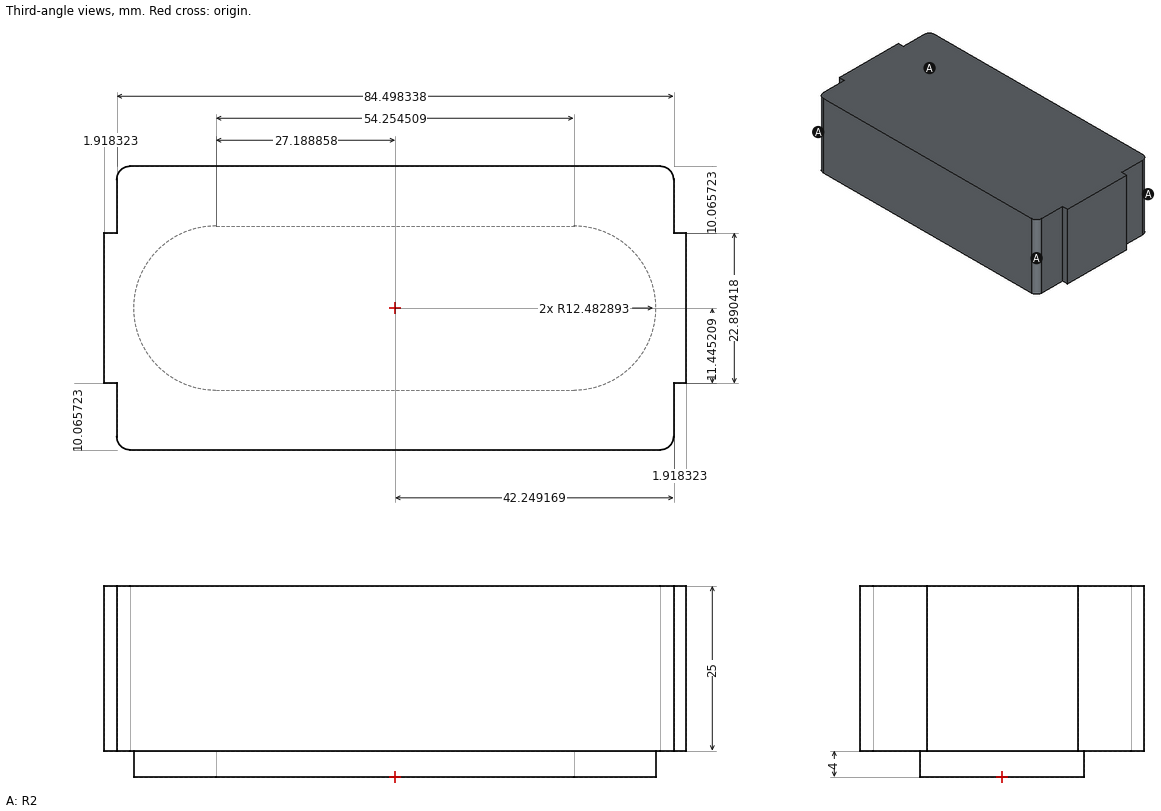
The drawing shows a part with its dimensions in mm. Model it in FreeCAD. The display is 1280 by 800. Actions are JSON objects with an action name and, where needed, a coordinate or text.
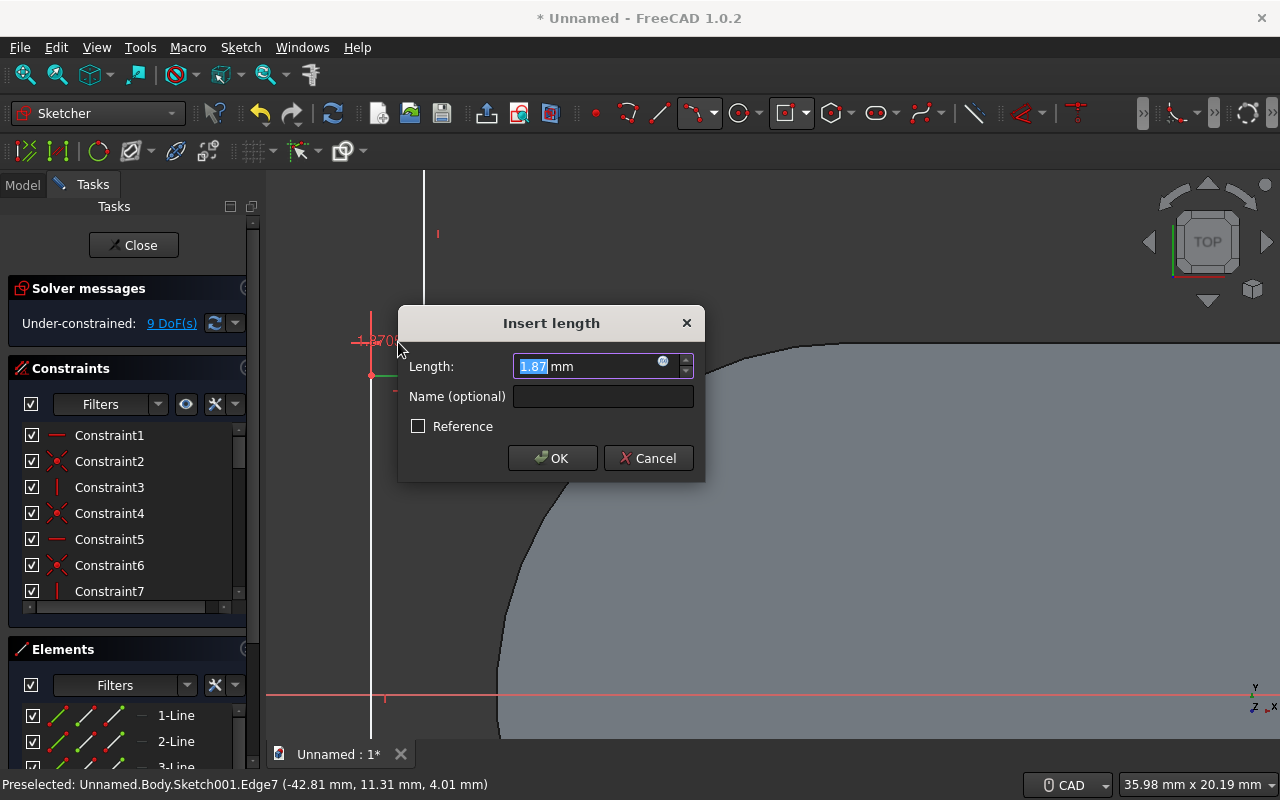
{"action": "type", "text": "1.918323"}
{"action": "key", "text": "Return"}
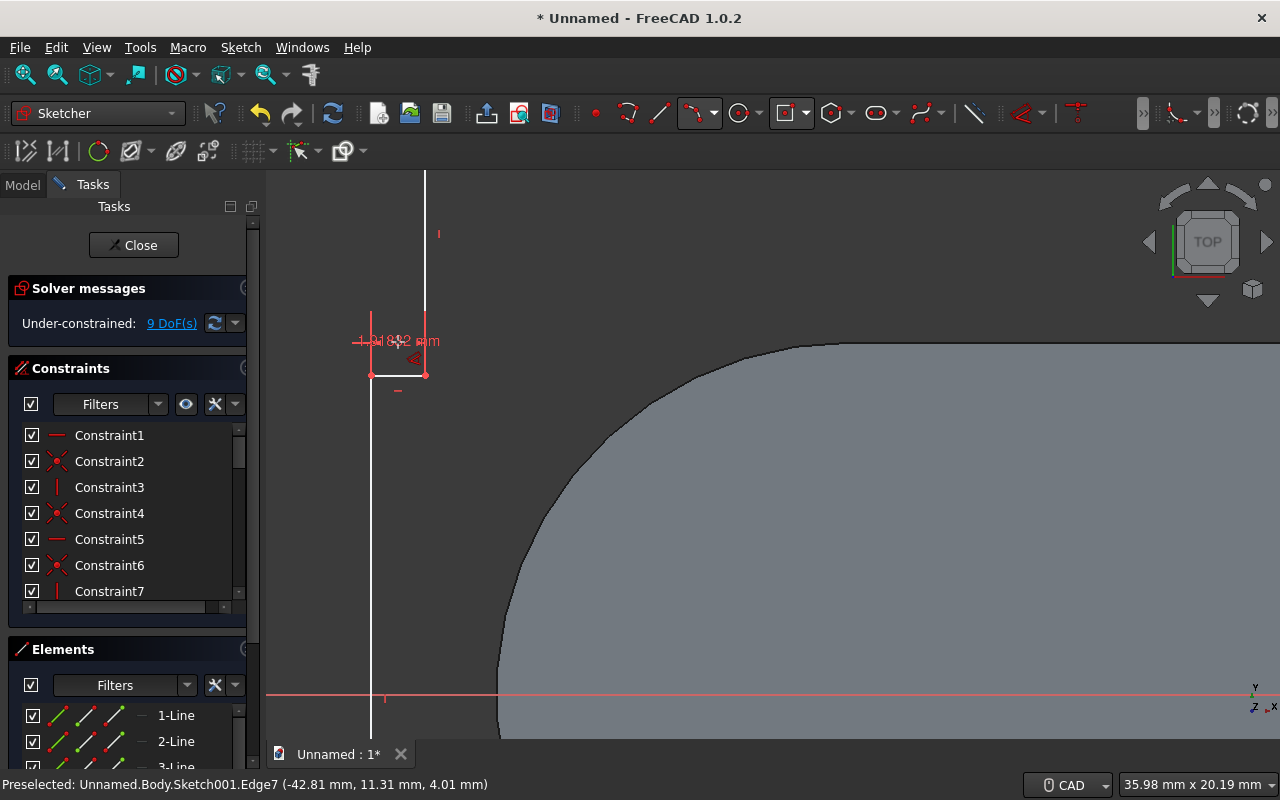
{"action": "scroll", "coordinate": [407, 376], "scroll_direction": "down", "scroll_amount": 7}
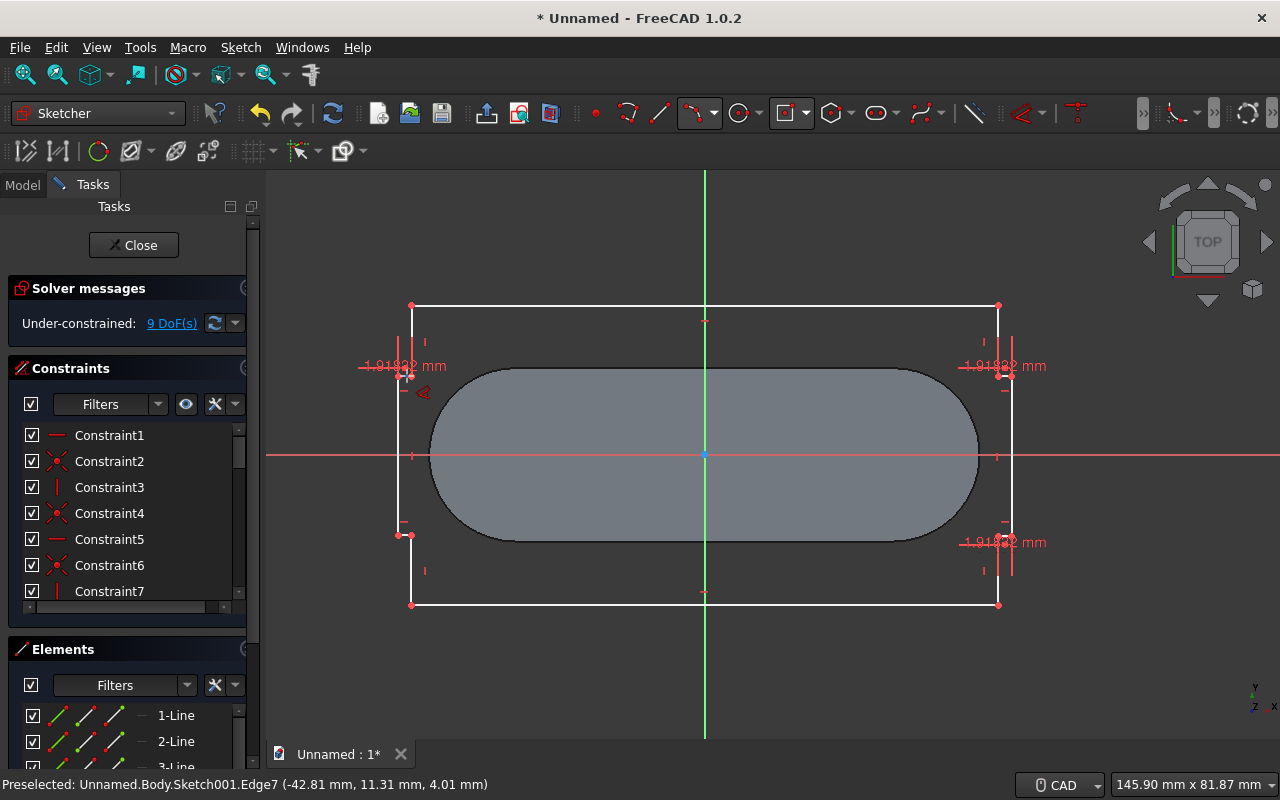
{"action": "scroll", "coordinate": [402, 535], "scroll_direction": "up", "scroll_amount": 7}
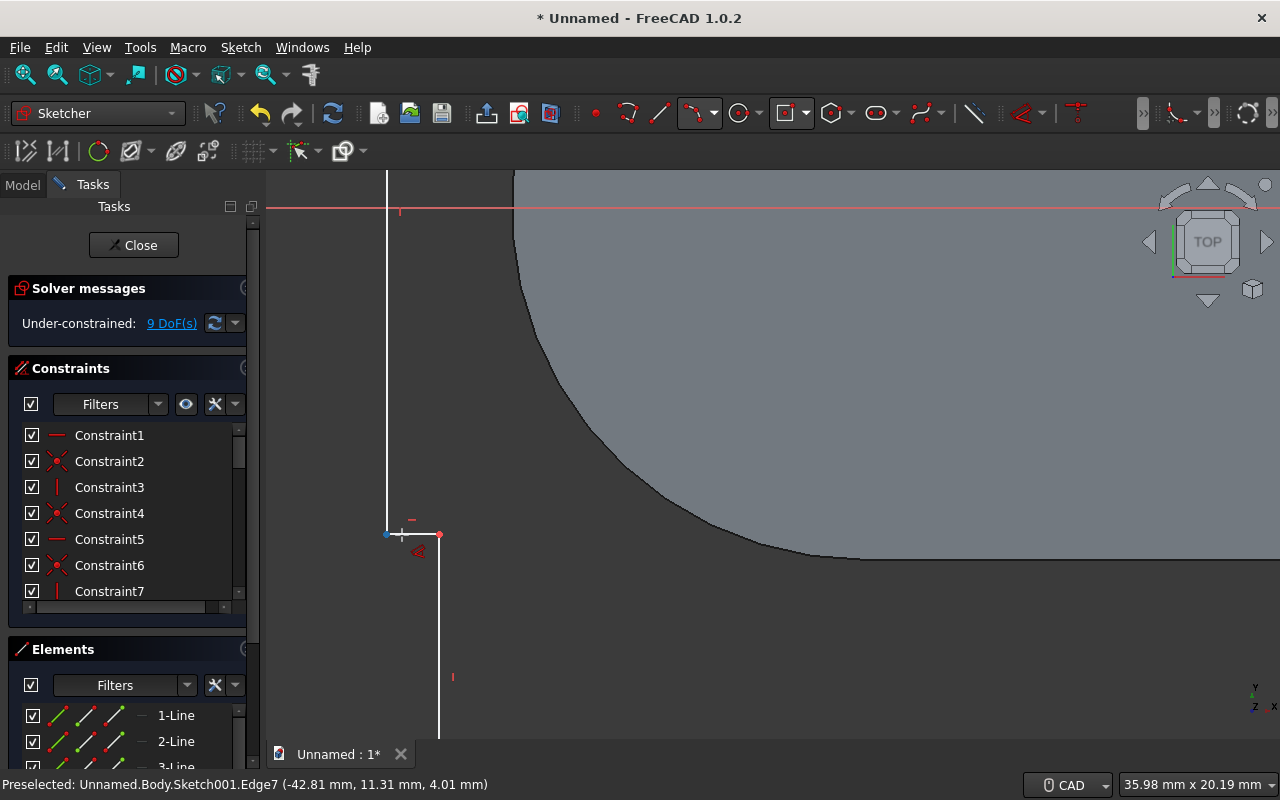
{"action": "left_click", "coordinate": [402, 534]}
{"action": "left_click", "coordinate": [413, 568]}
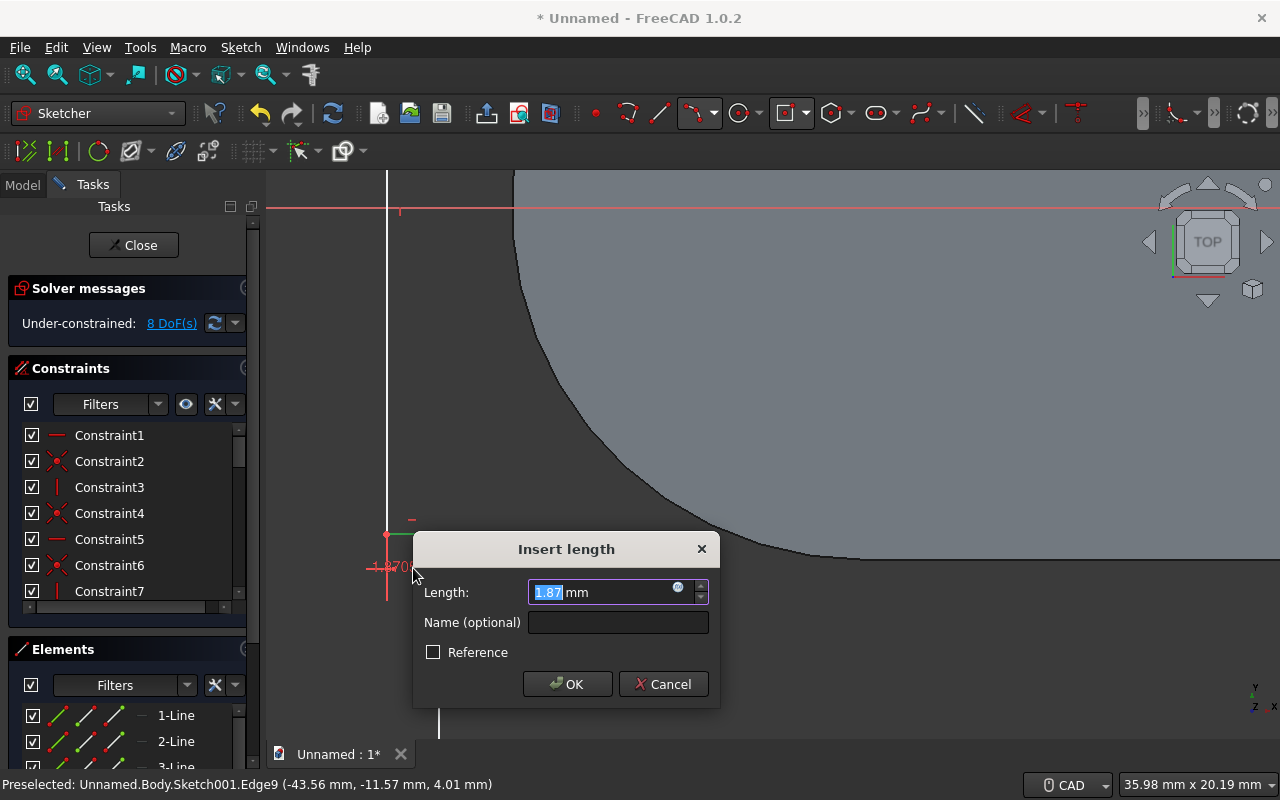
{"action": "type", "text": "1.918323"}
{"action": "key", "text": "Return"}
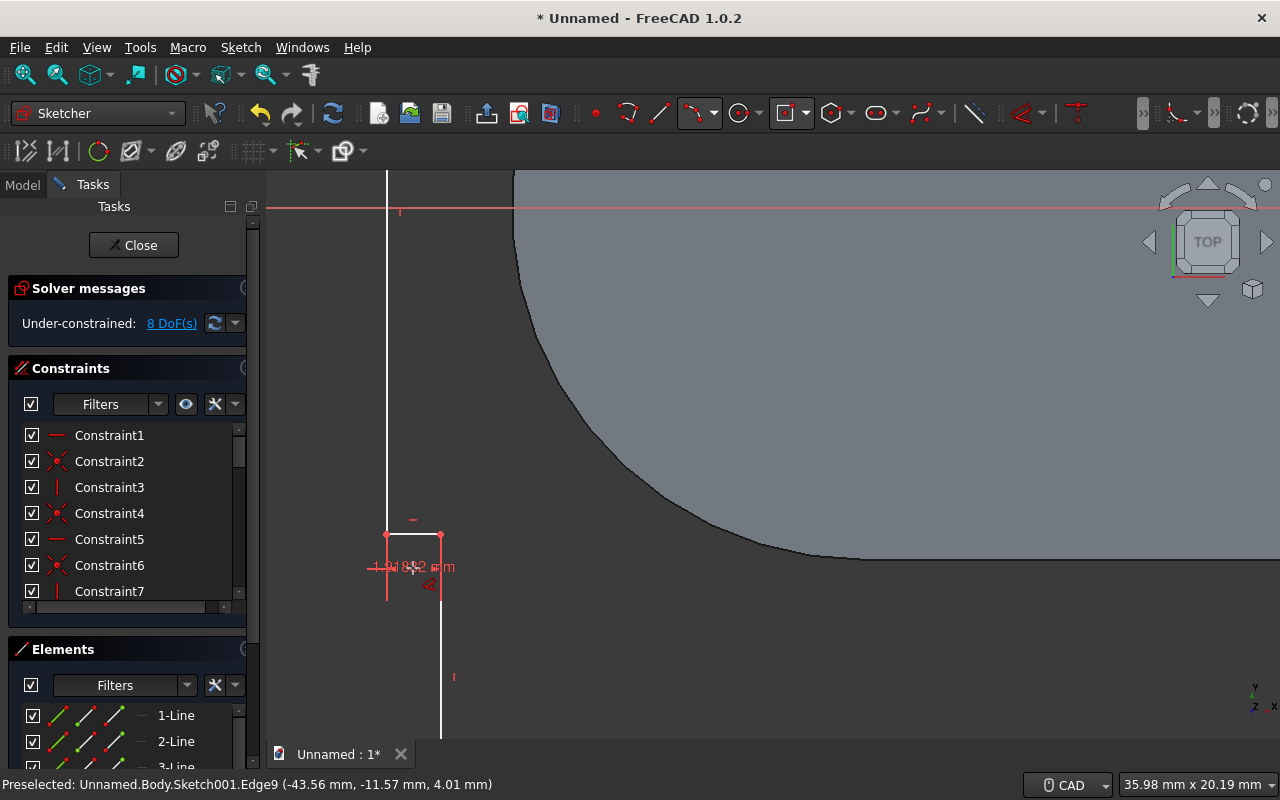
{"action": "scroll", "coordinate": [402, 535], "scroll_direction": "down", "scroll_amount": 7}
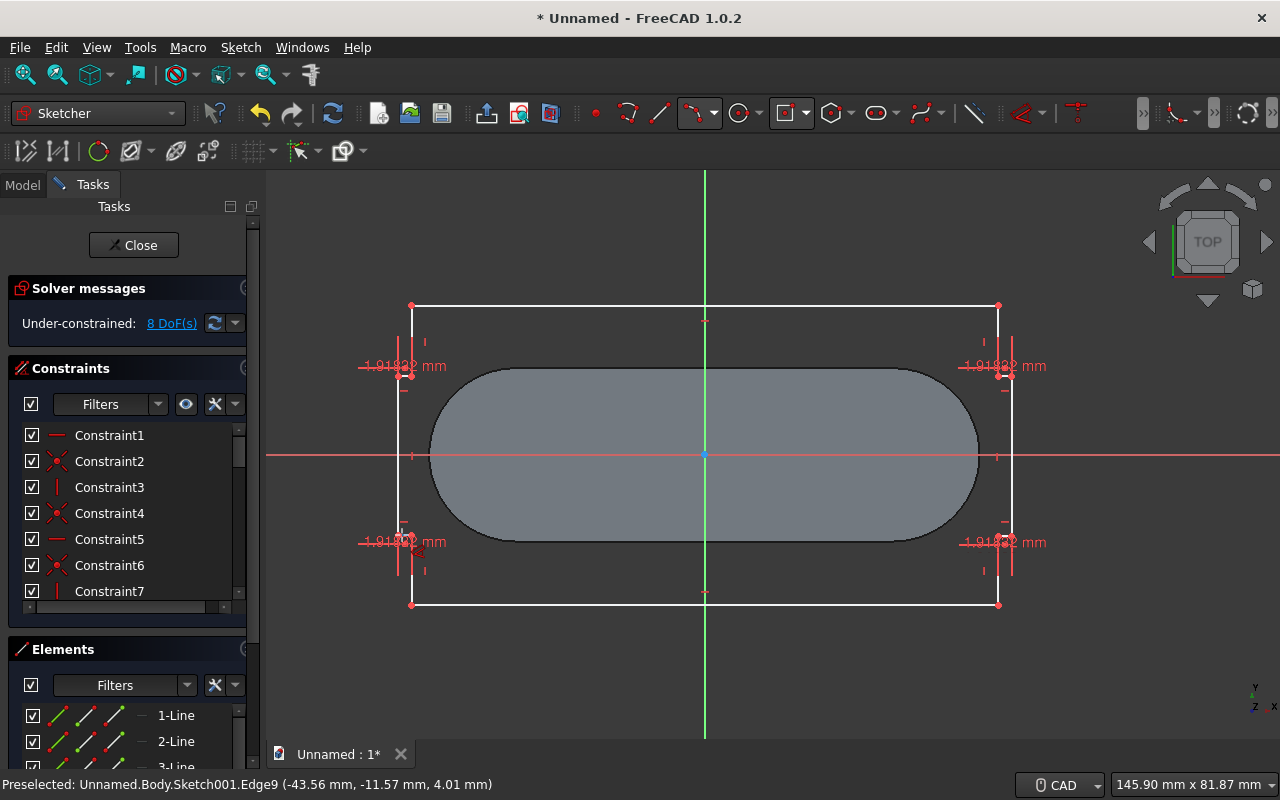
{"action": "left_click", "coordinate": [1012, 488]}
{"action": "left_click", "coordinate": [1046, 419]}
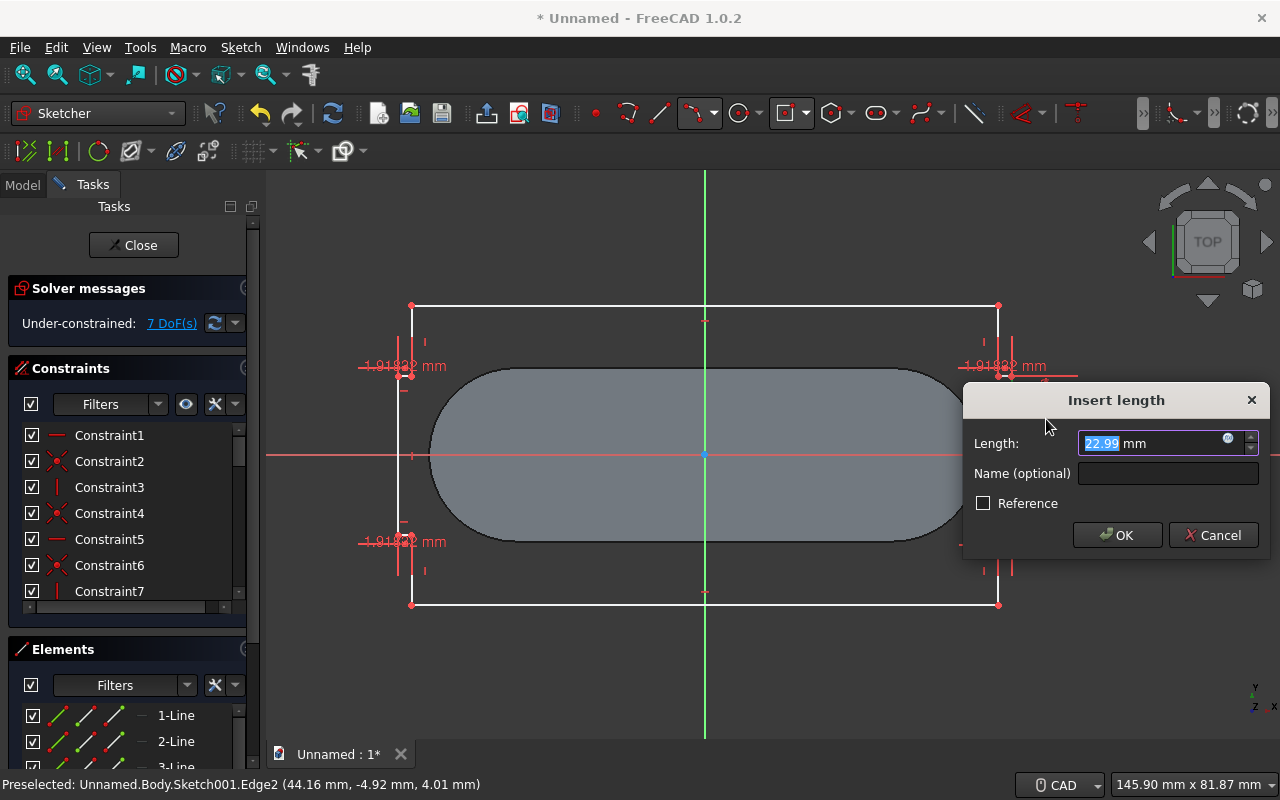
{"action": "type", "text": "22.890418"}
{"action": "key", "text": "Return"}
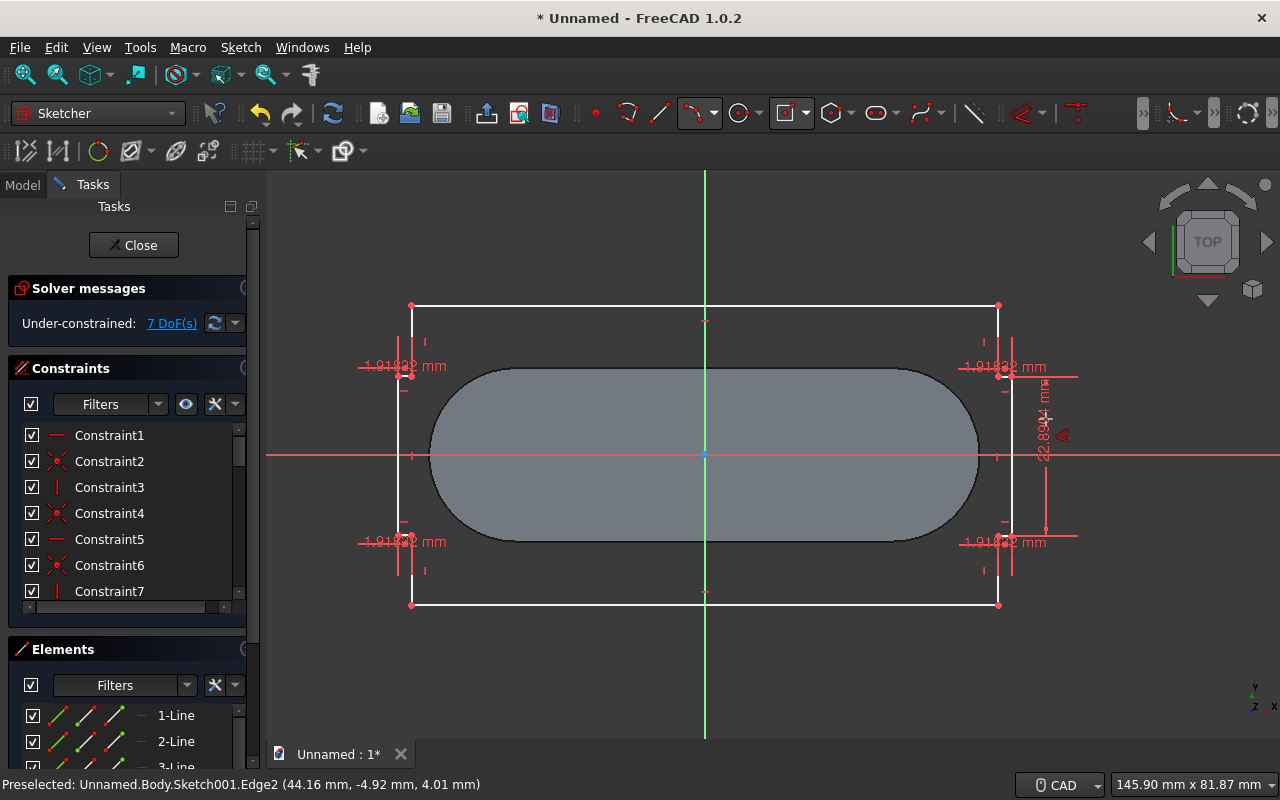
{"action": "left_click", "coordinate": [998, 356]}
{"action": "left_click", "coordinate": [1032, 341]}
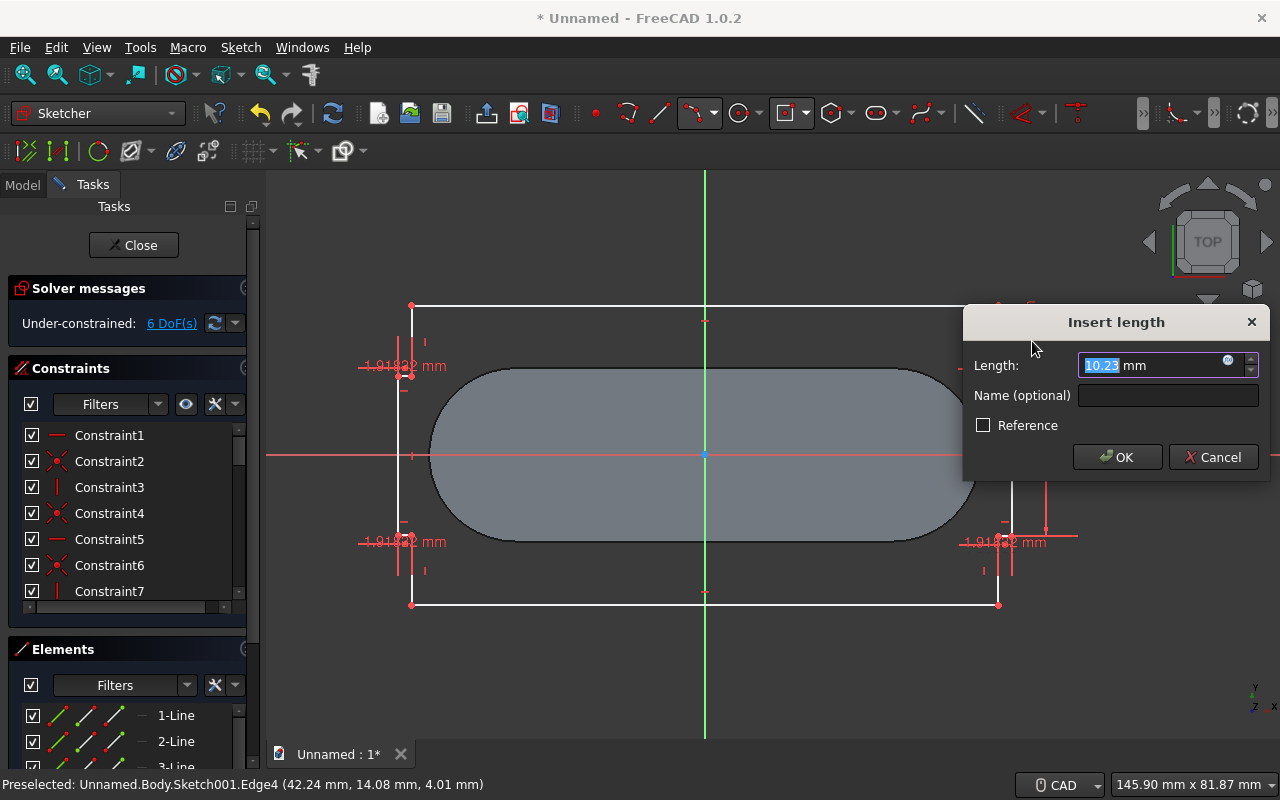
{"action": "type", "text": "10.065723"}
{"action": "key", "text": "Return"}